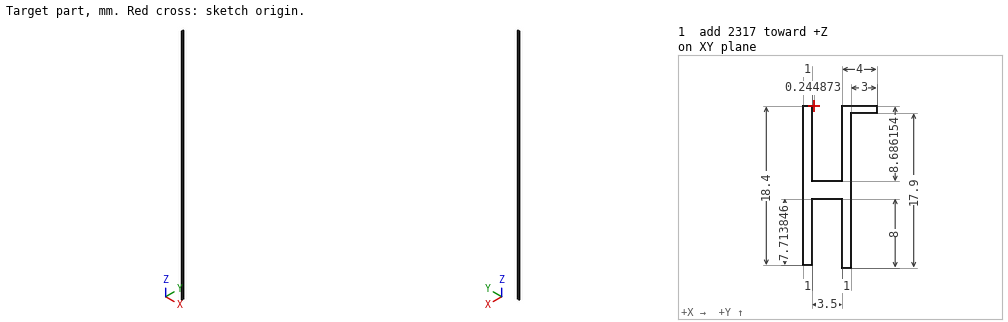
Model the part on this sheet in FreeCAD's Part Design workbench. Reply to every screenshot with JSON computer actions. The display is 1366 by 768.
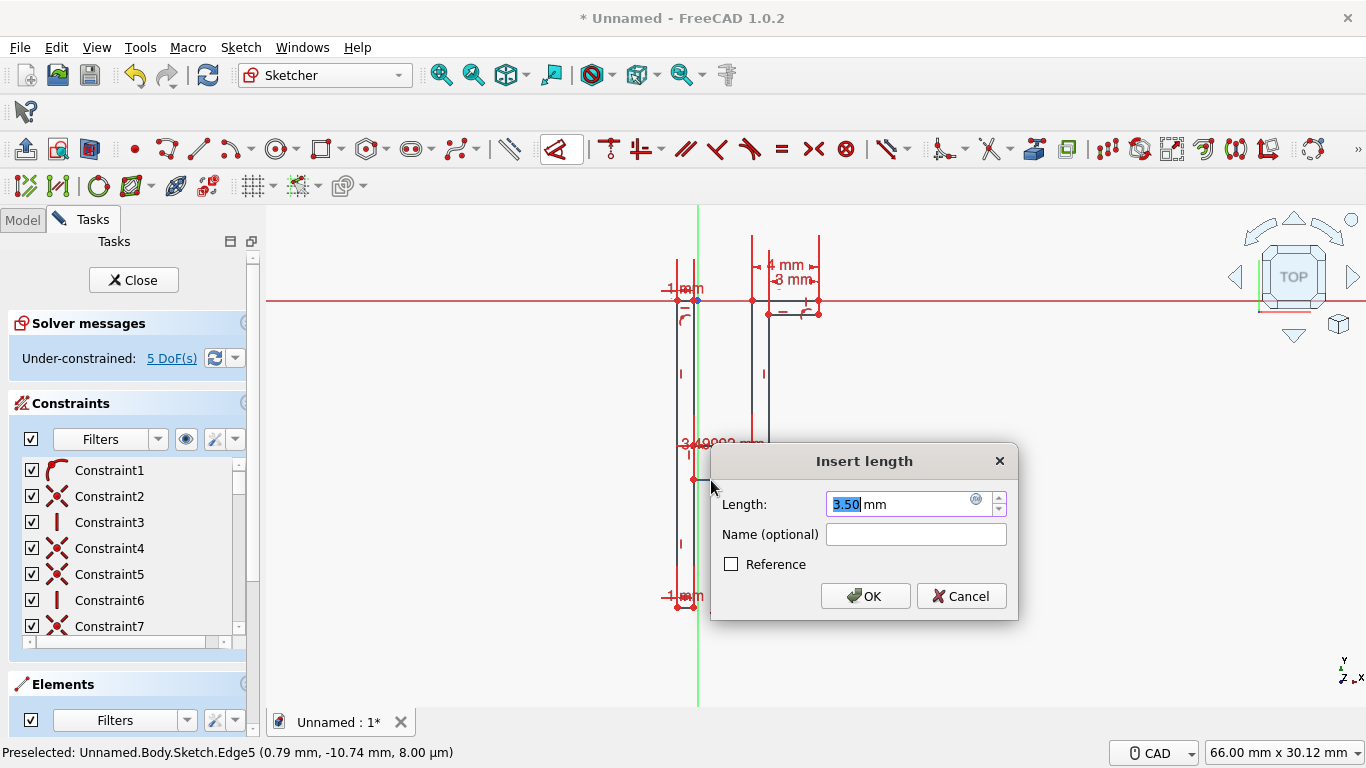
{"action": "type", "text": "3.5"}
{"action": "key", "text": "Return"}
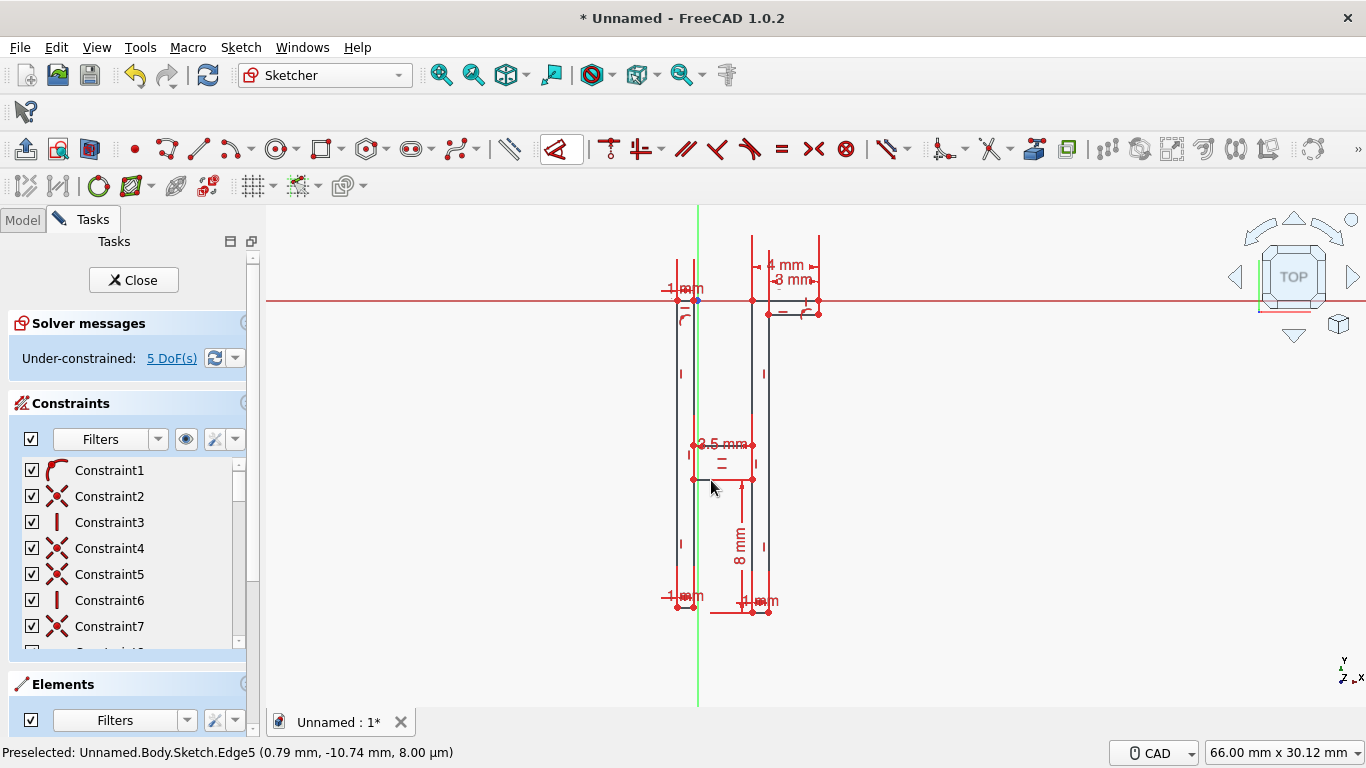
{"action": "left_click", "coordinate": [677, 393]}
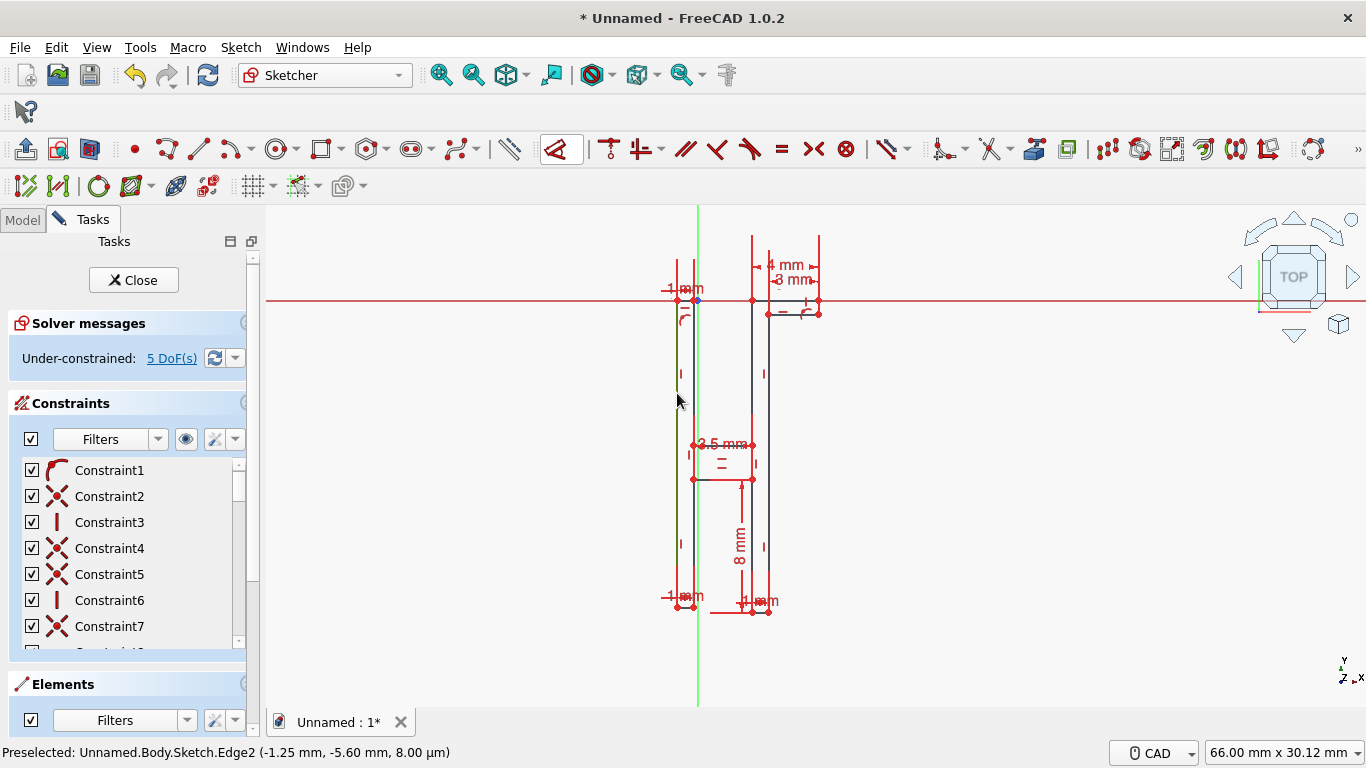
{"action": "key", "text": "i"}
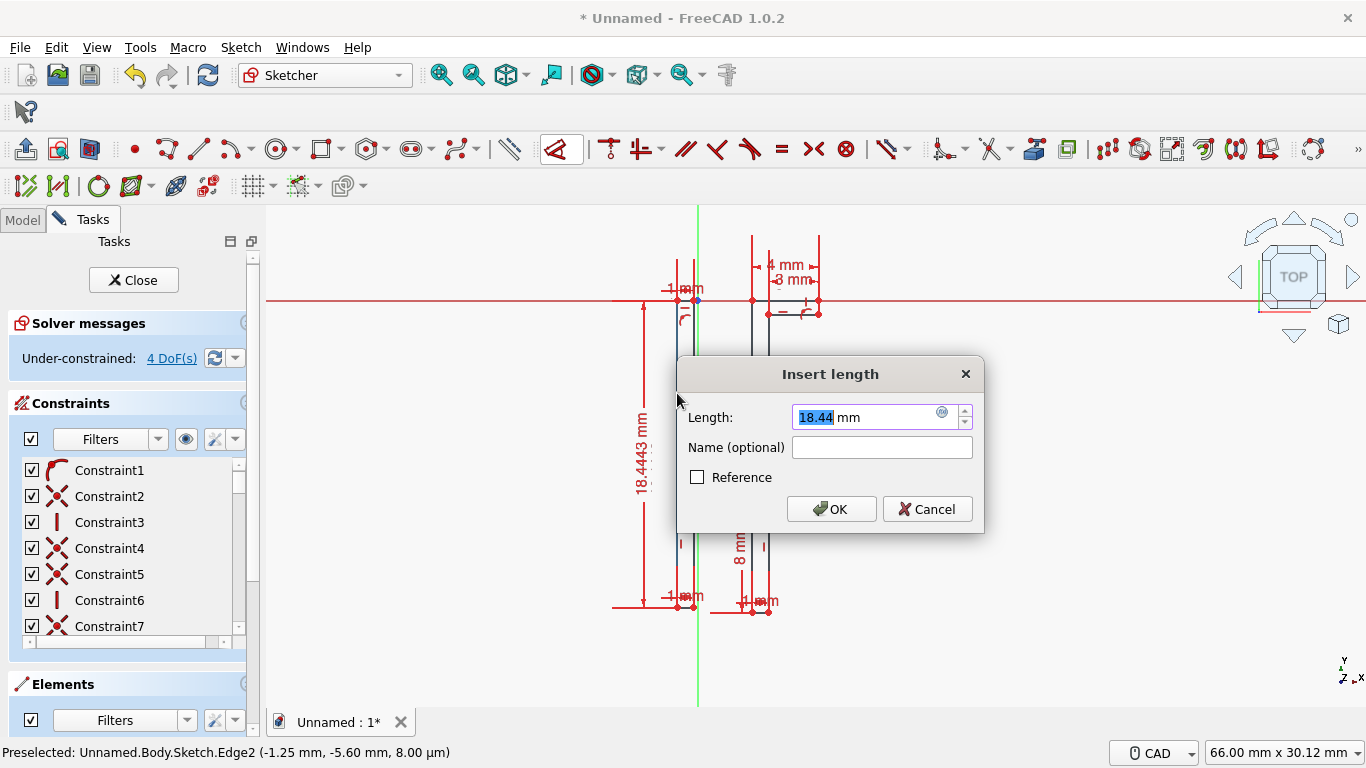
{"action": "type", "text": "18.4"}
{"action": "key", "text": "Return"}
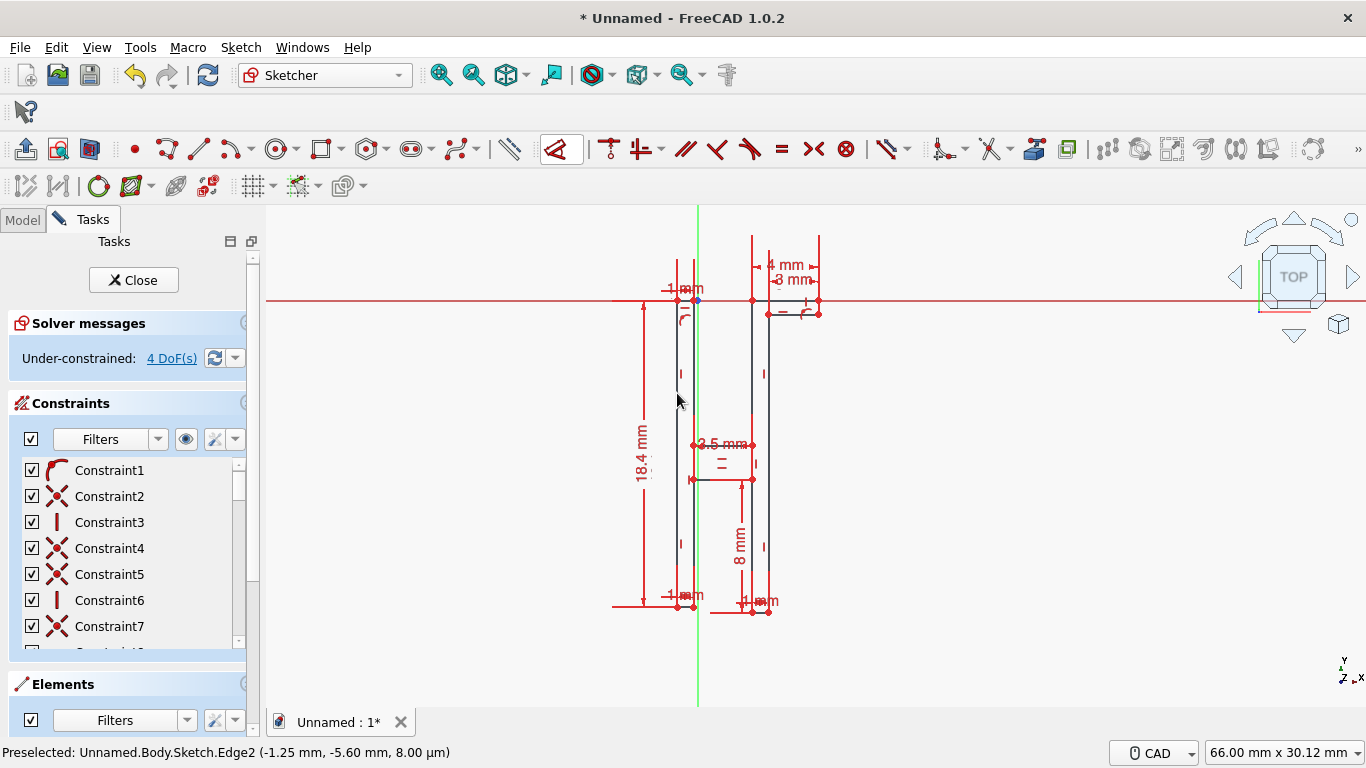
{"action": "left_click", "coordinate": [769, 524]}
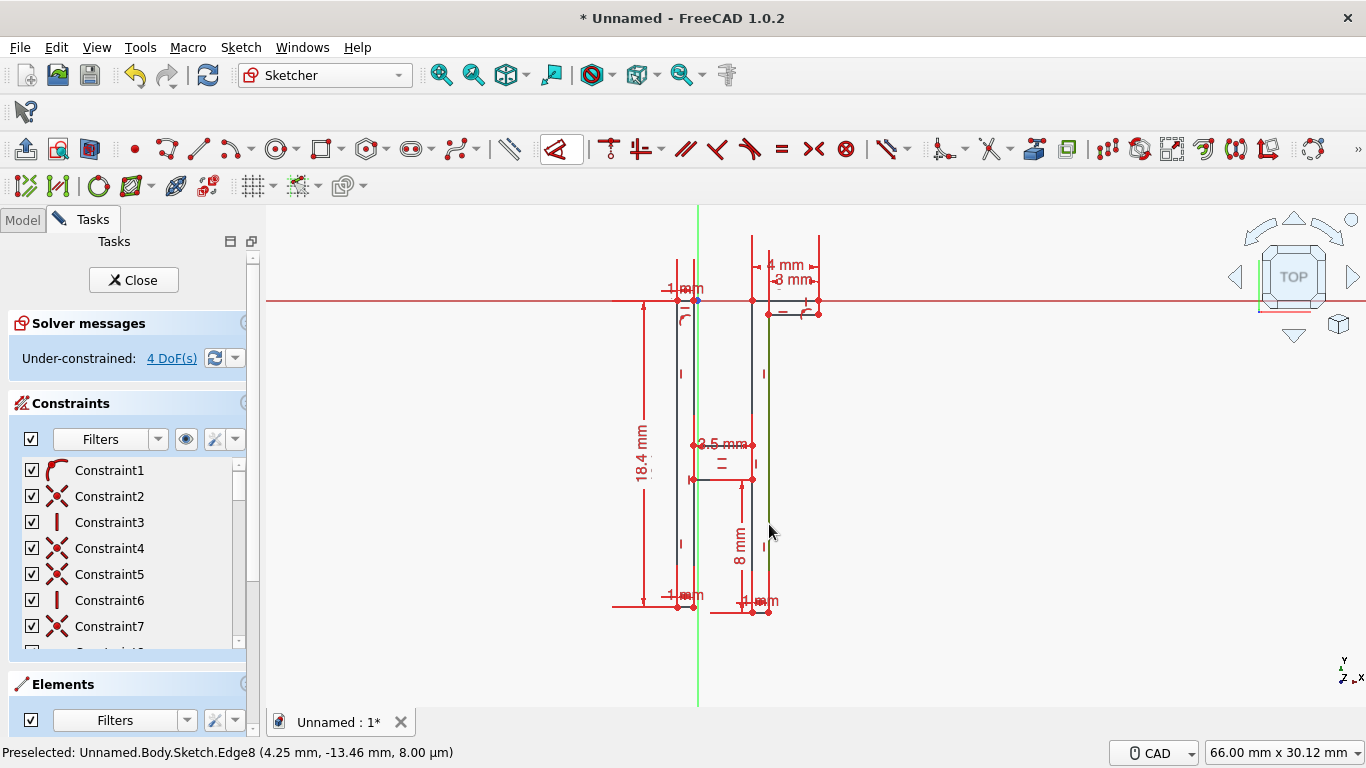
{"action": "key", "text": "i"}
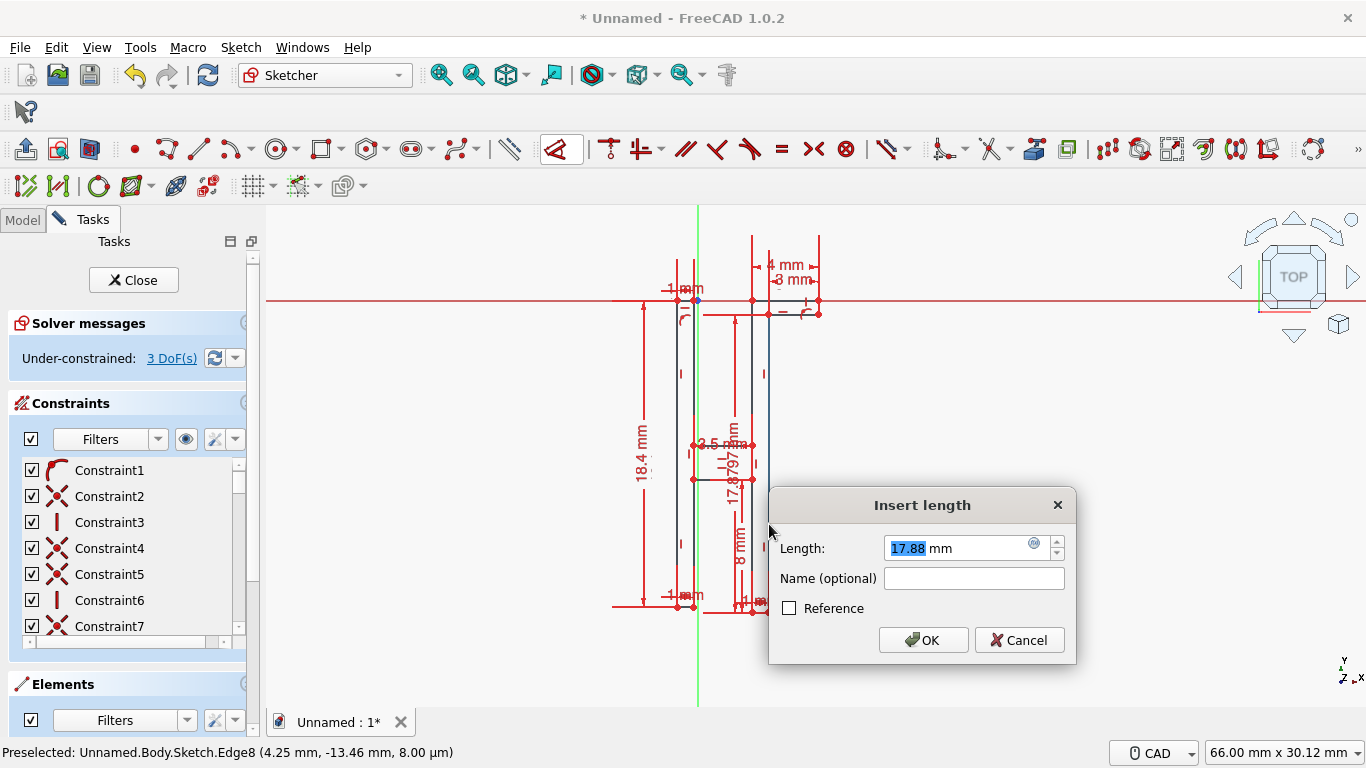
{"action": "type", "text": "17.9"}
{"action": "key", "text": "Return"}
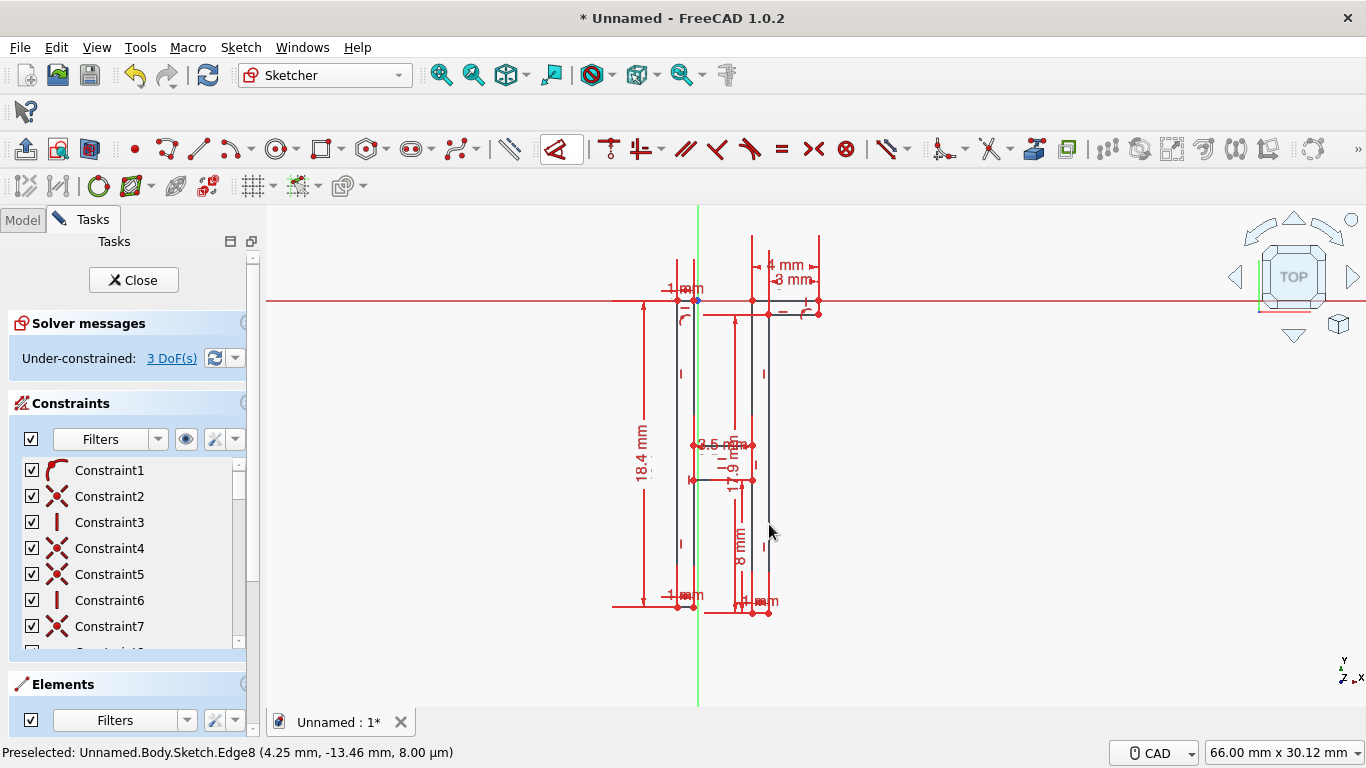
{"action": "scroll", "coordinate": [694, 569], "scroll_direction": "up", "scroll_amount": 6}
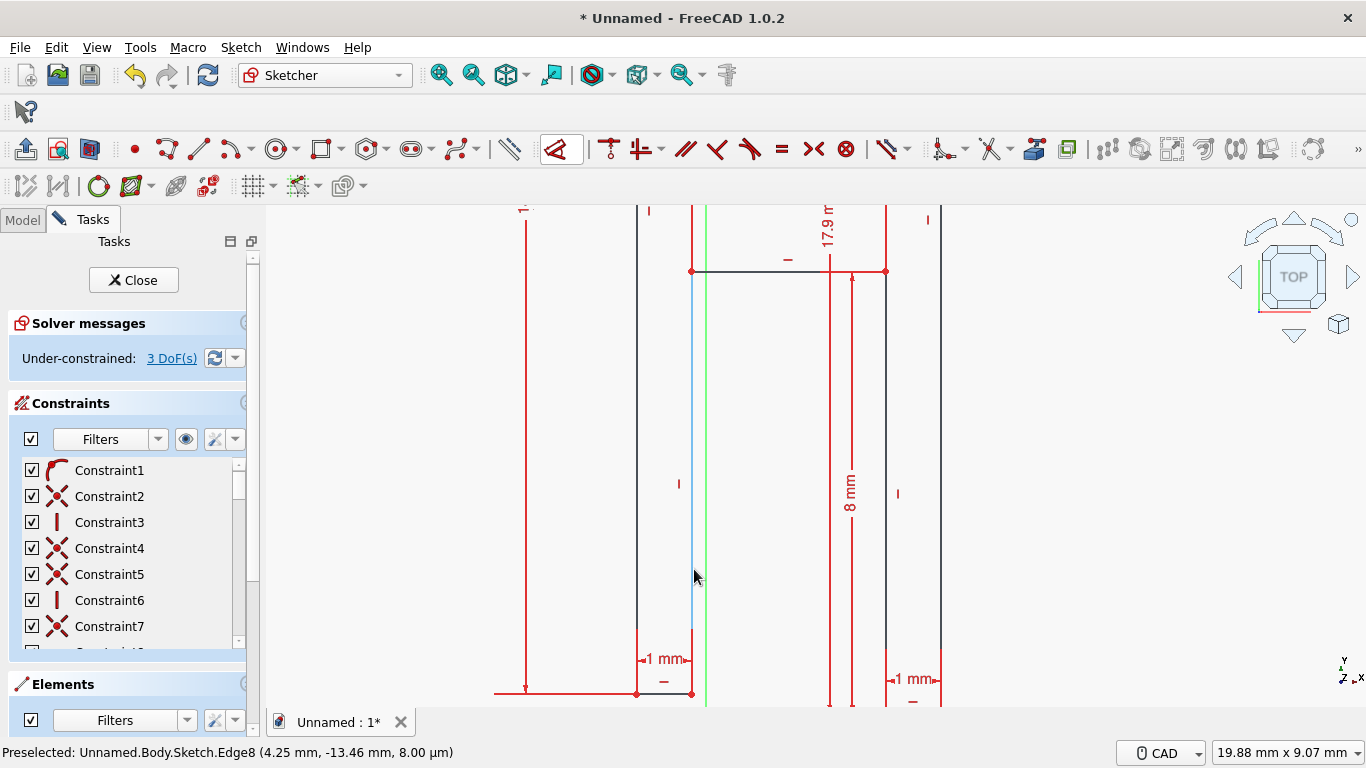
{"action": "left_click", "coordinate": [692, 568]}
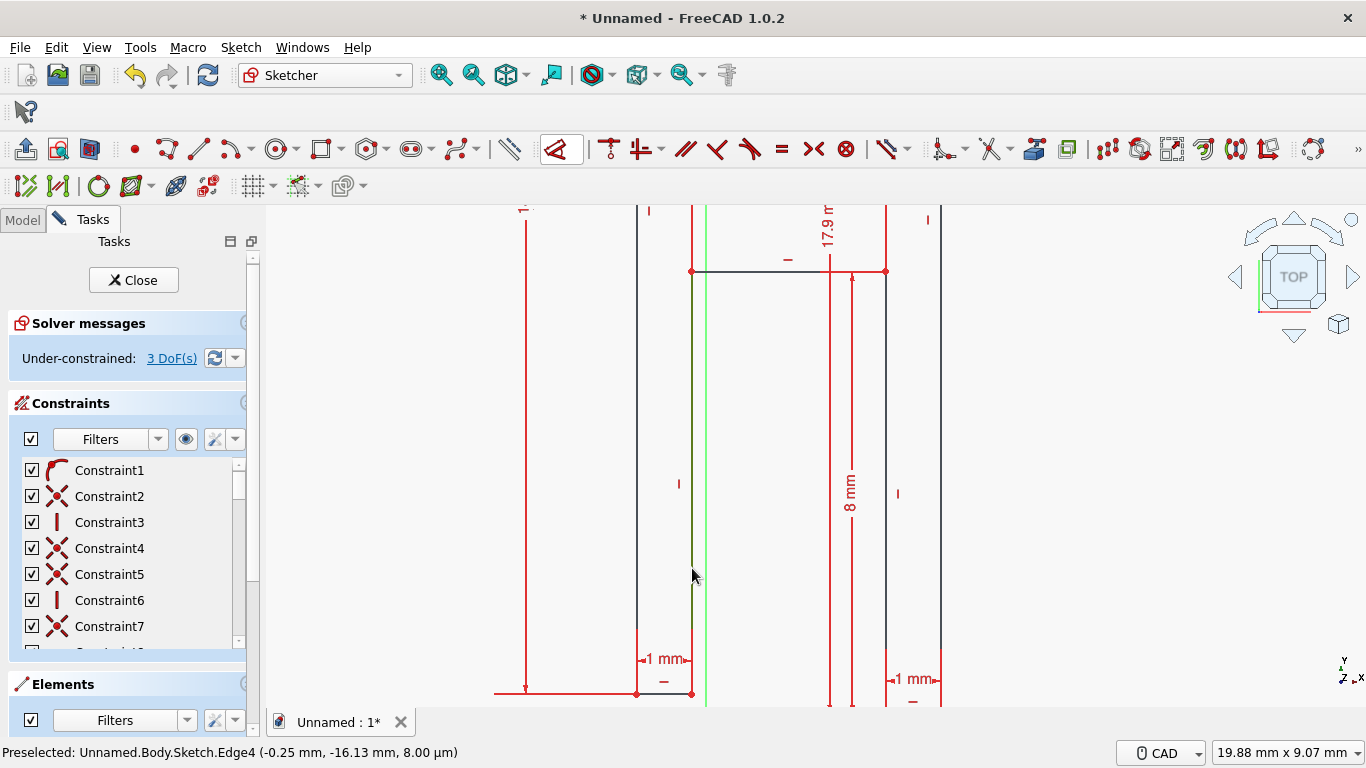
{"action": "key", "text": "i"}